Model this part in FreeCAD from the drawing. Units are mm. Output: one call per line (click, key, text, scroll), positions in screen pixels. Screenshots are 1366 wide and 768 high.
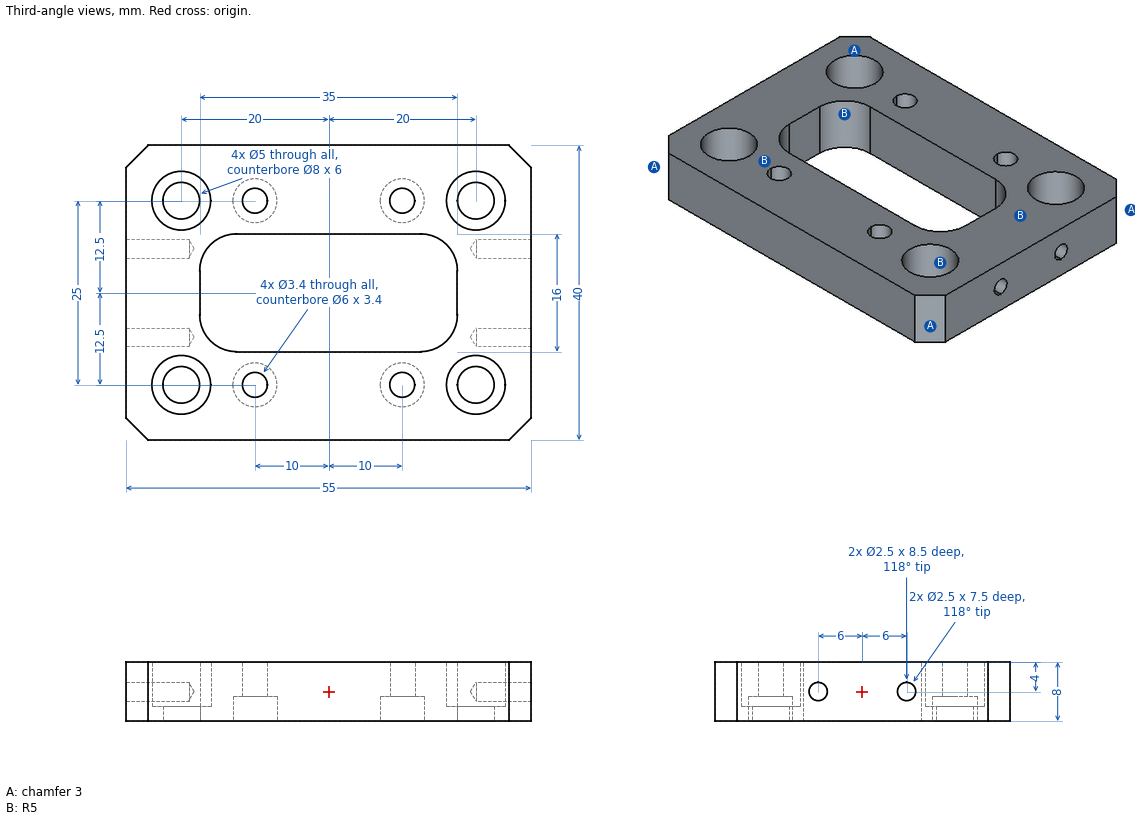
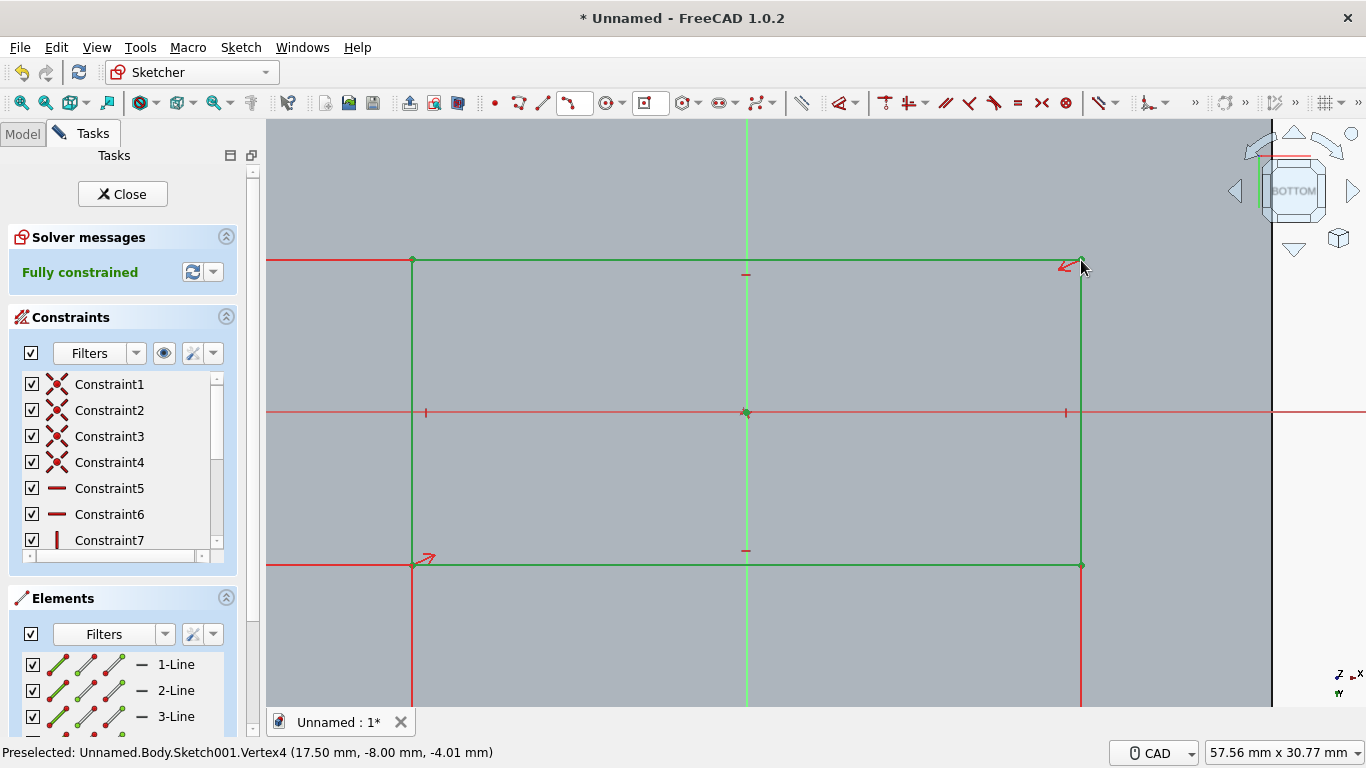
click(123, 194)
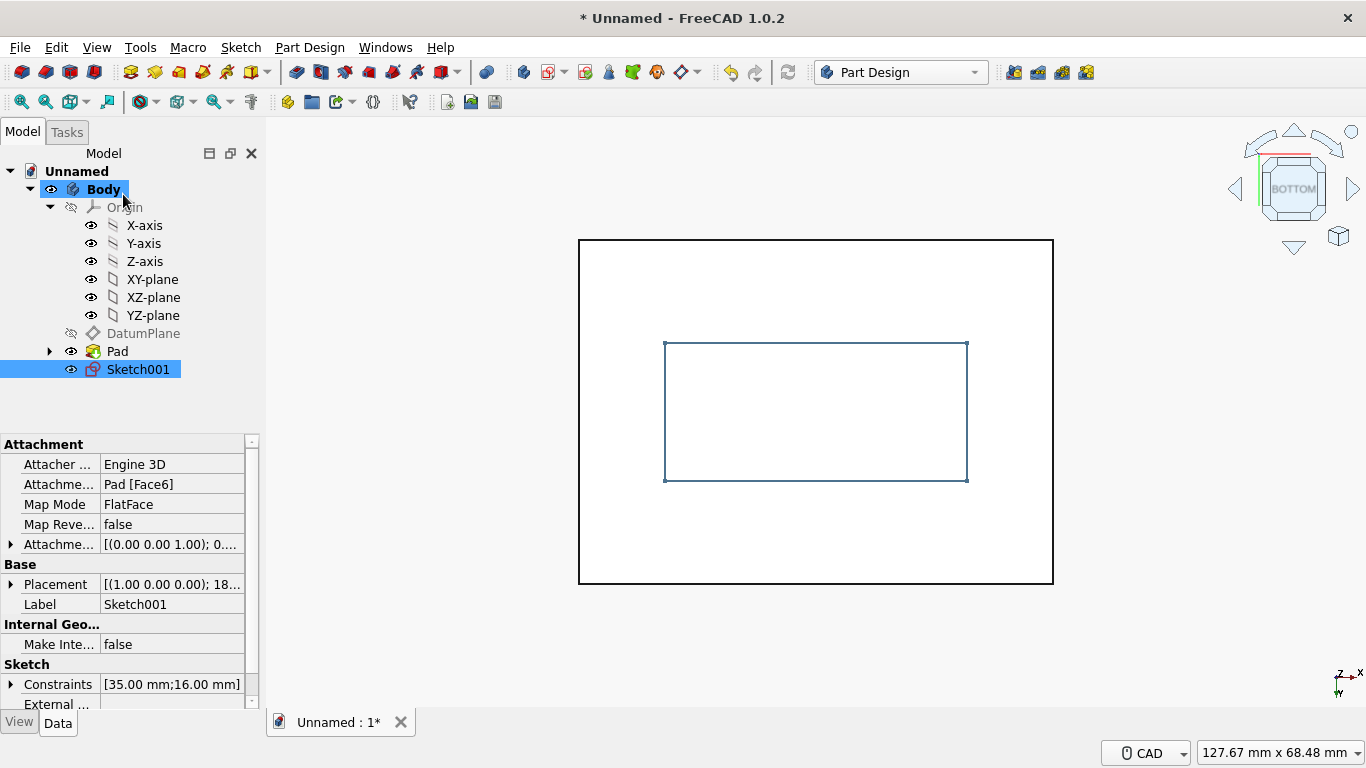
click(298, 72)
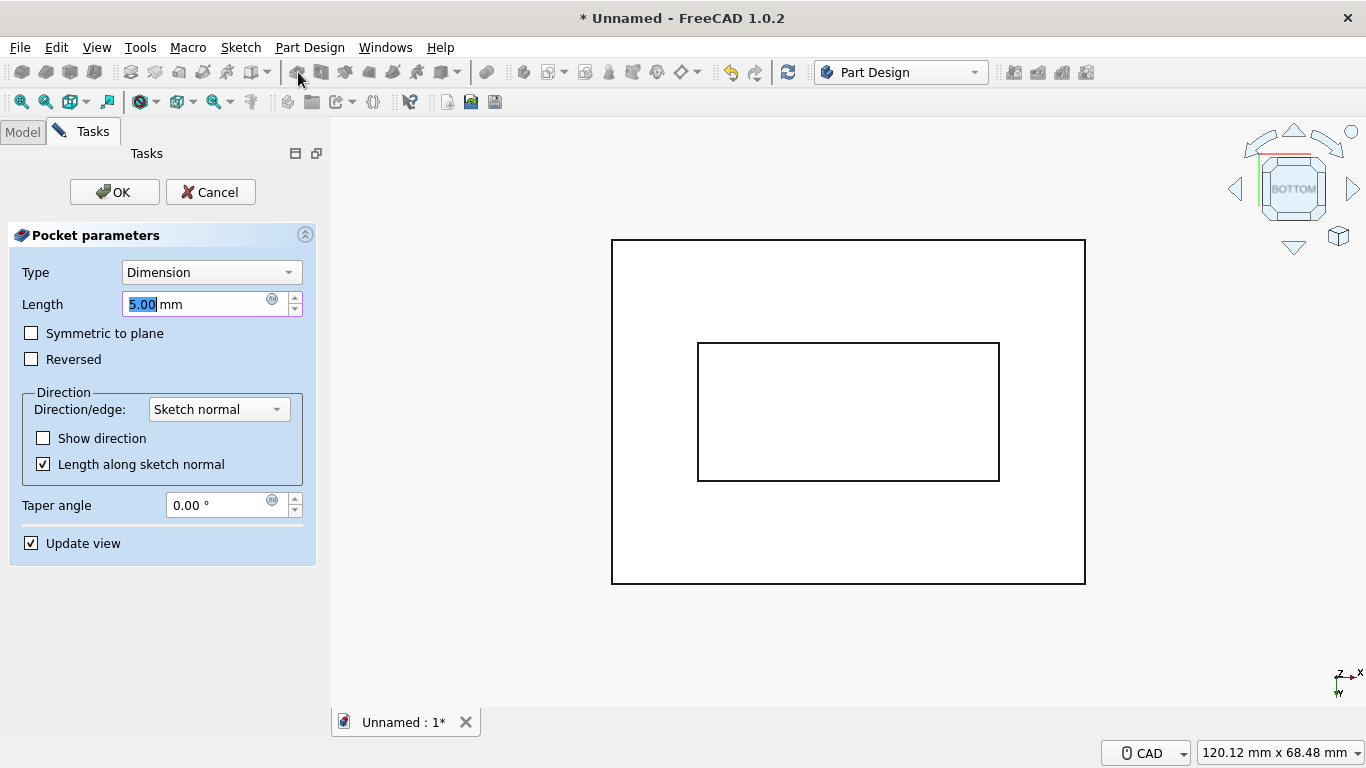
click(212, 272)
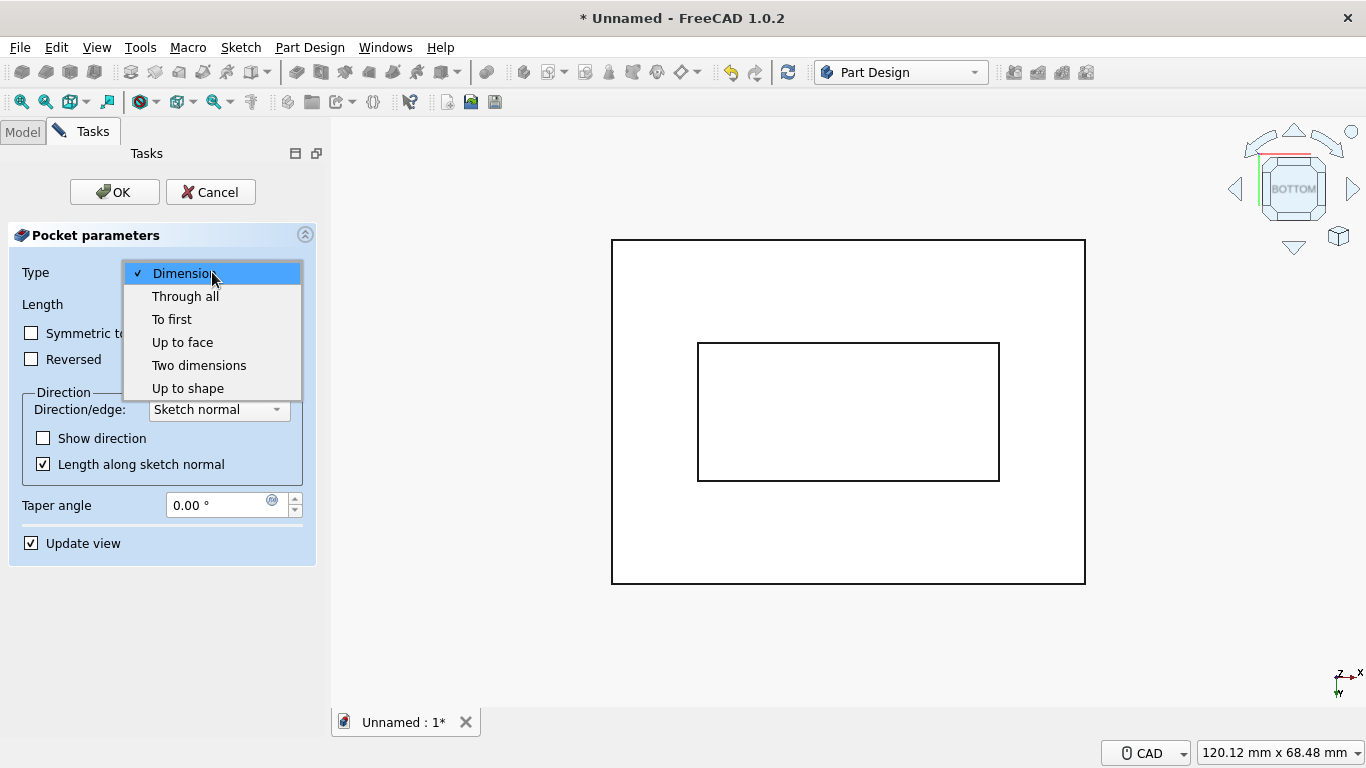
click(212, 296)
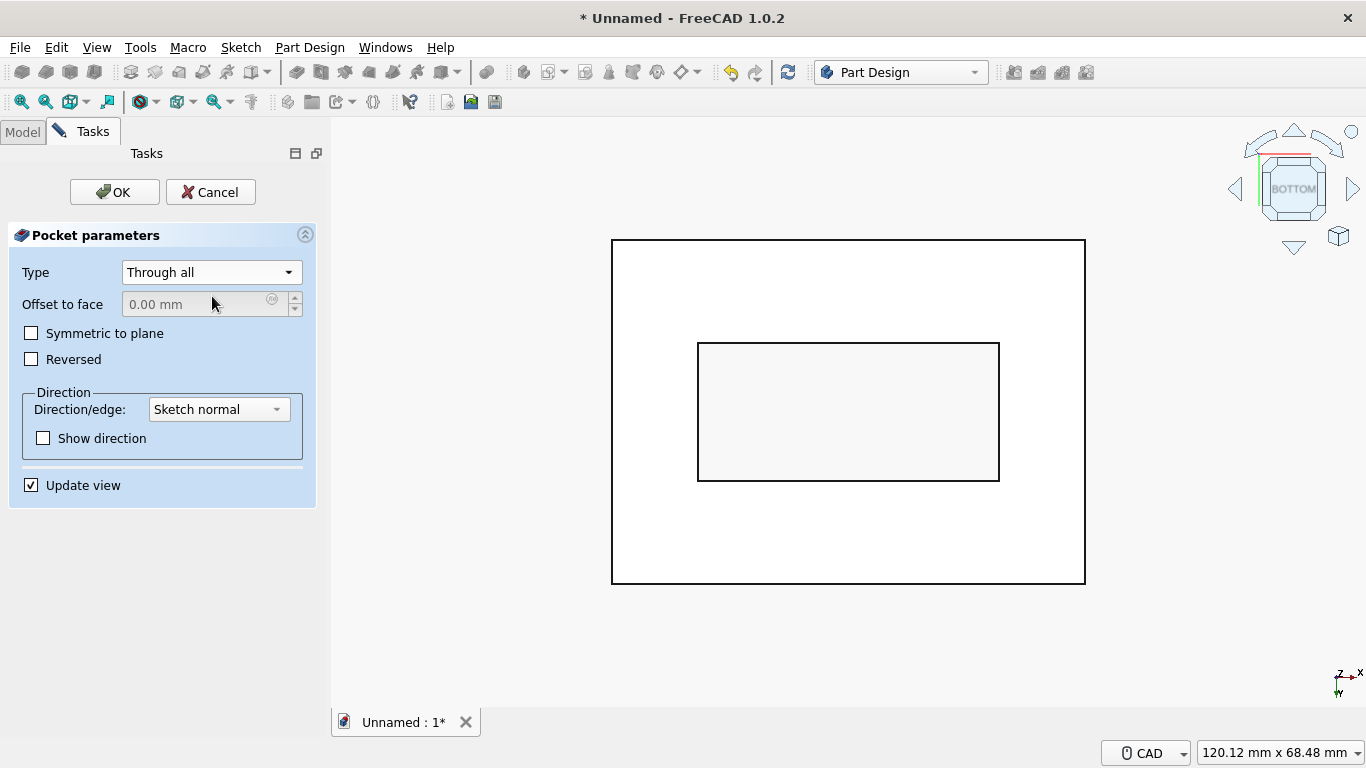
click(115, 192)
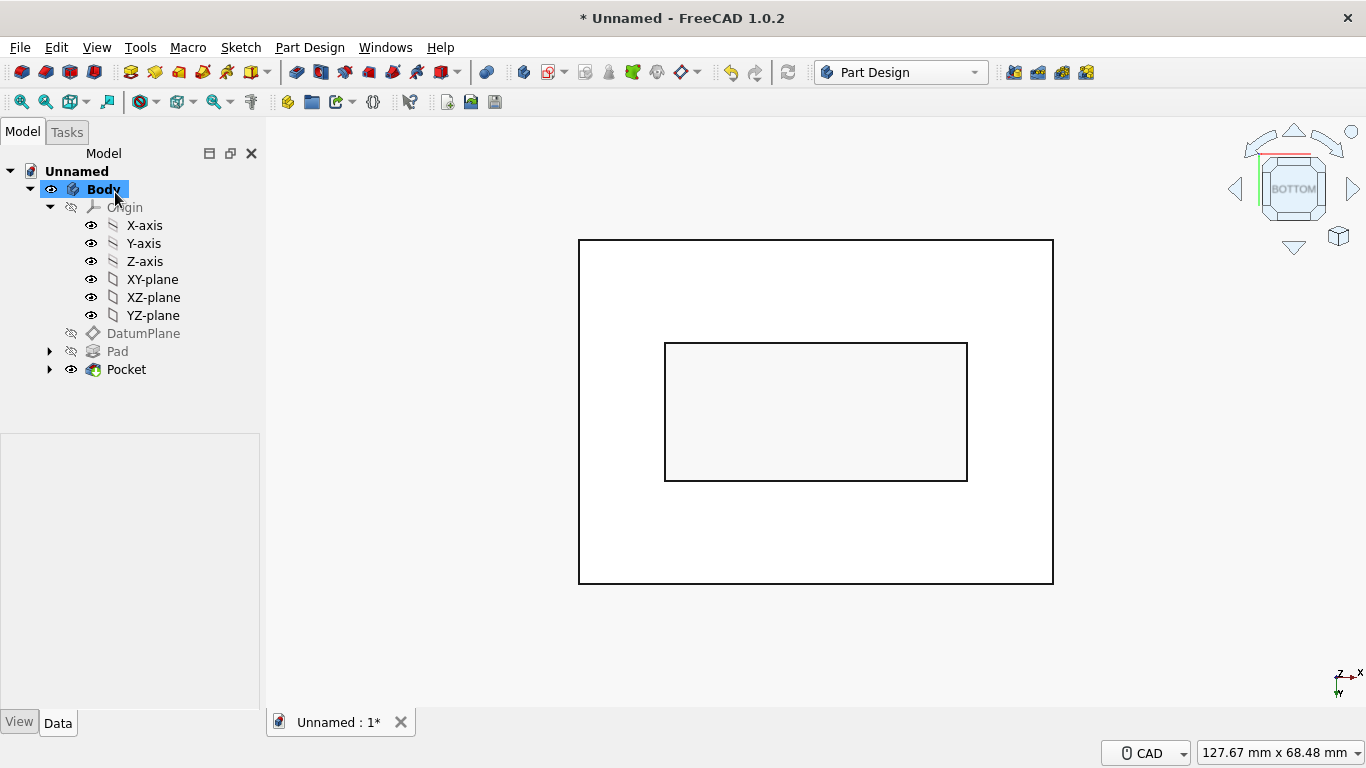
click(1019, 509)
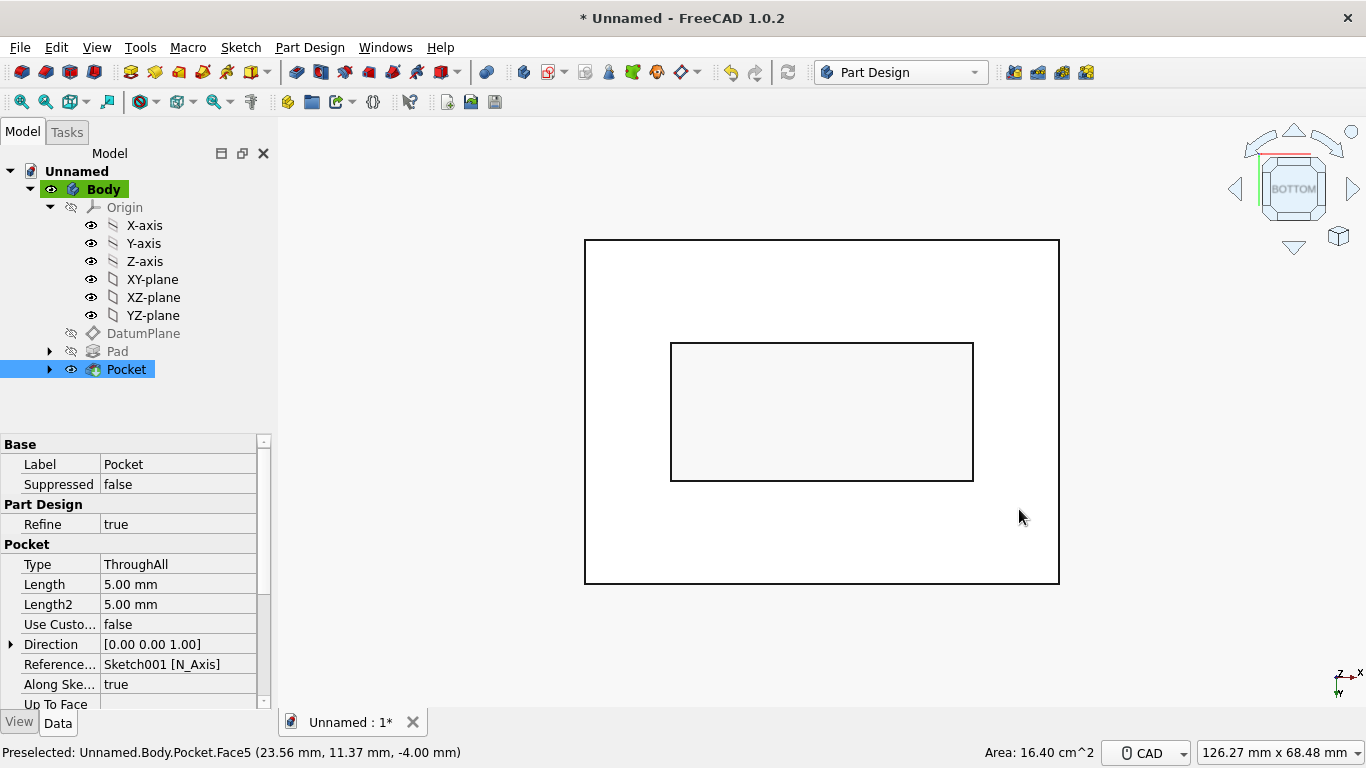
click(548, 72)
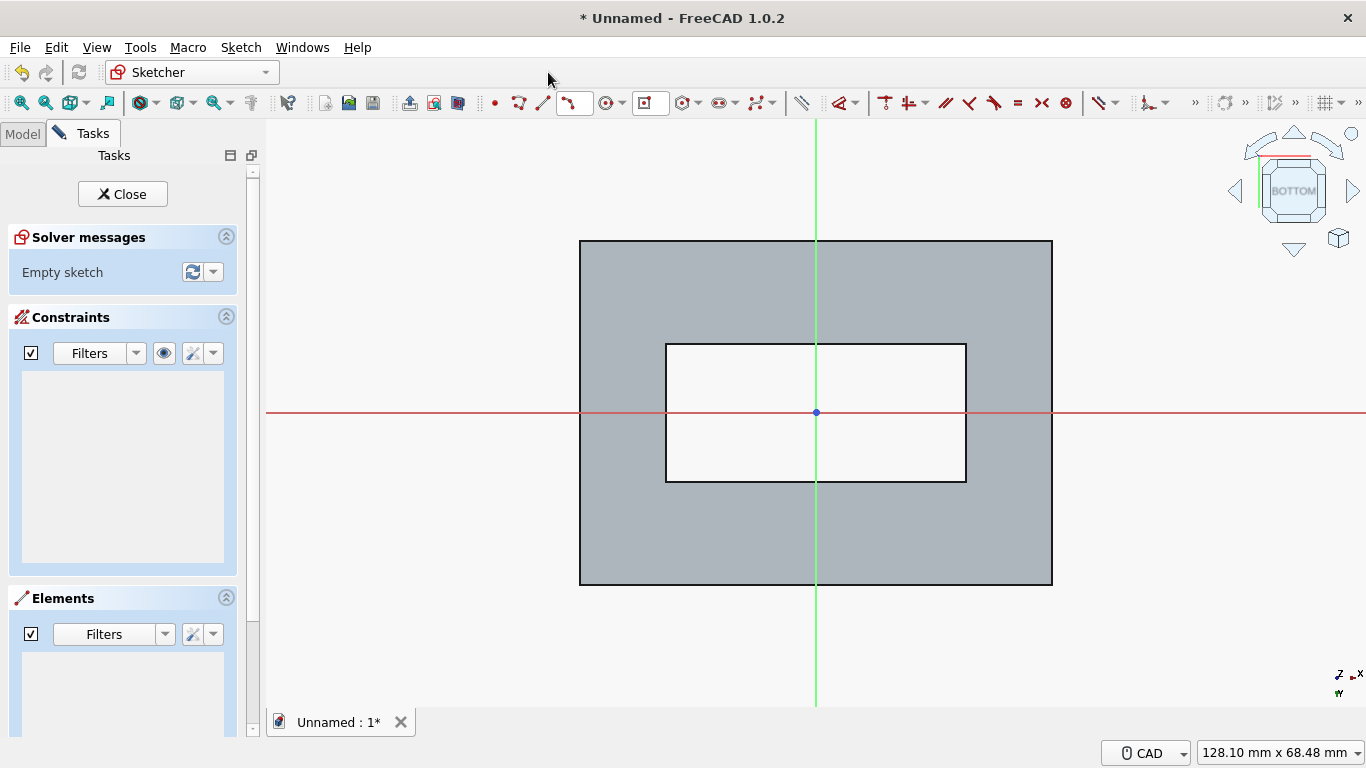
scroll(955, 413, up, 2)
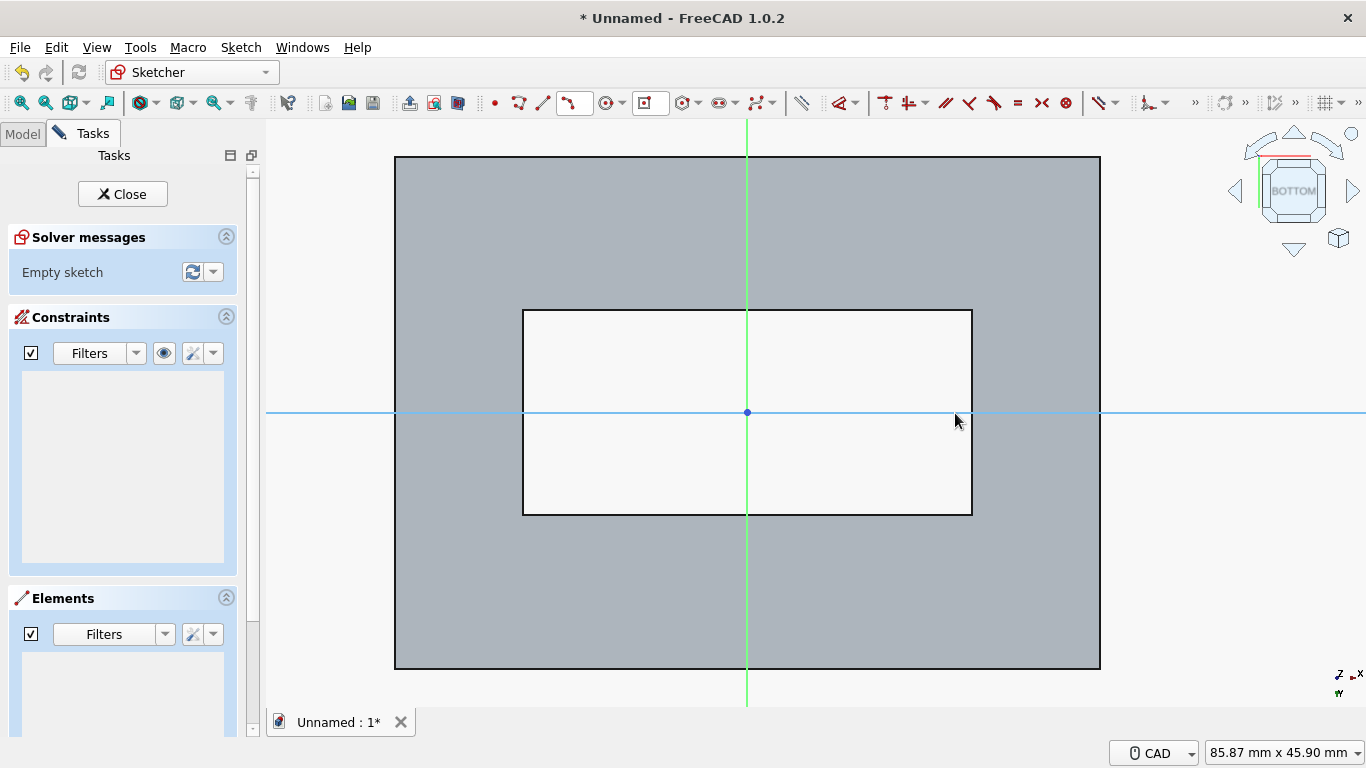
click(606, 104)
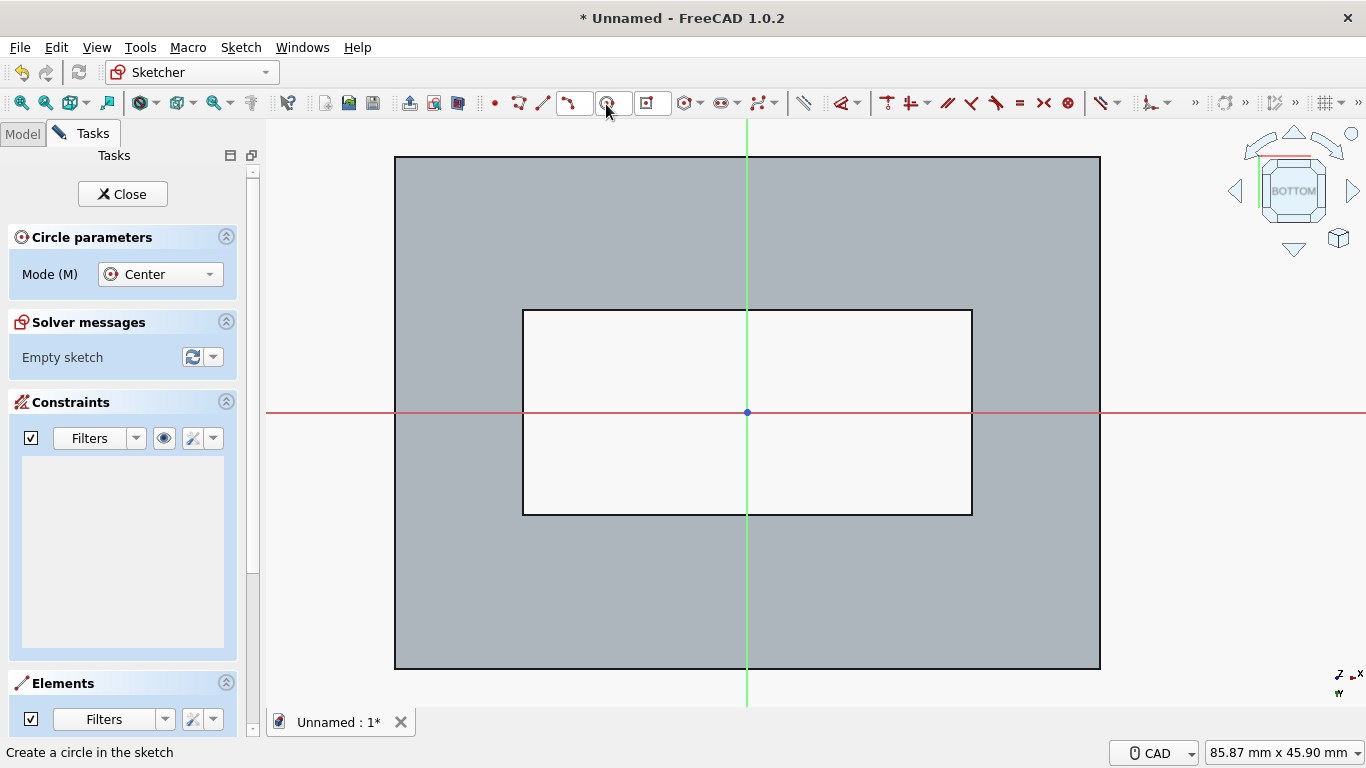
click(619, 253)
move(635, 237)